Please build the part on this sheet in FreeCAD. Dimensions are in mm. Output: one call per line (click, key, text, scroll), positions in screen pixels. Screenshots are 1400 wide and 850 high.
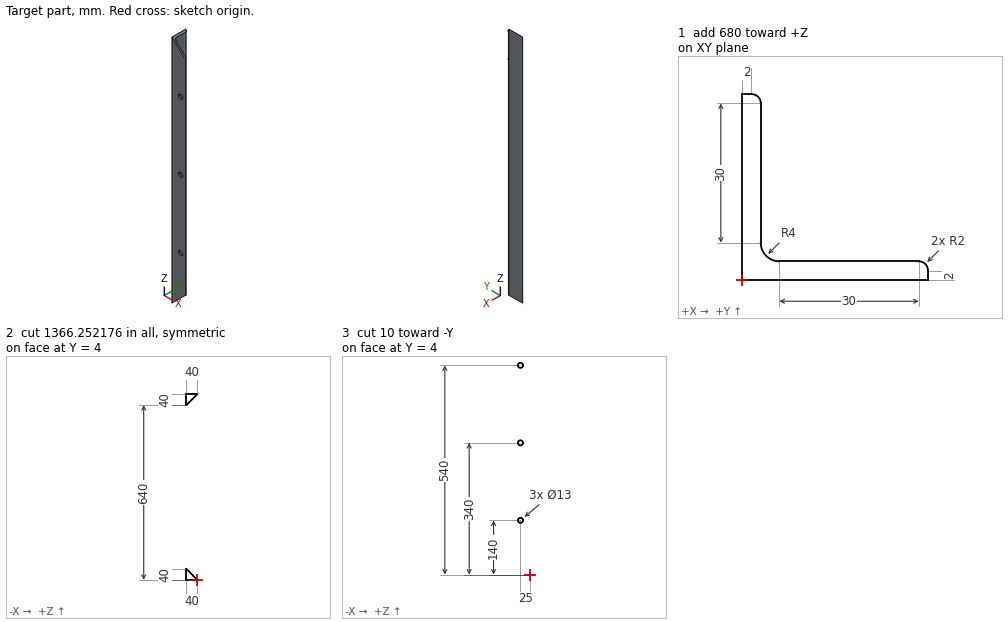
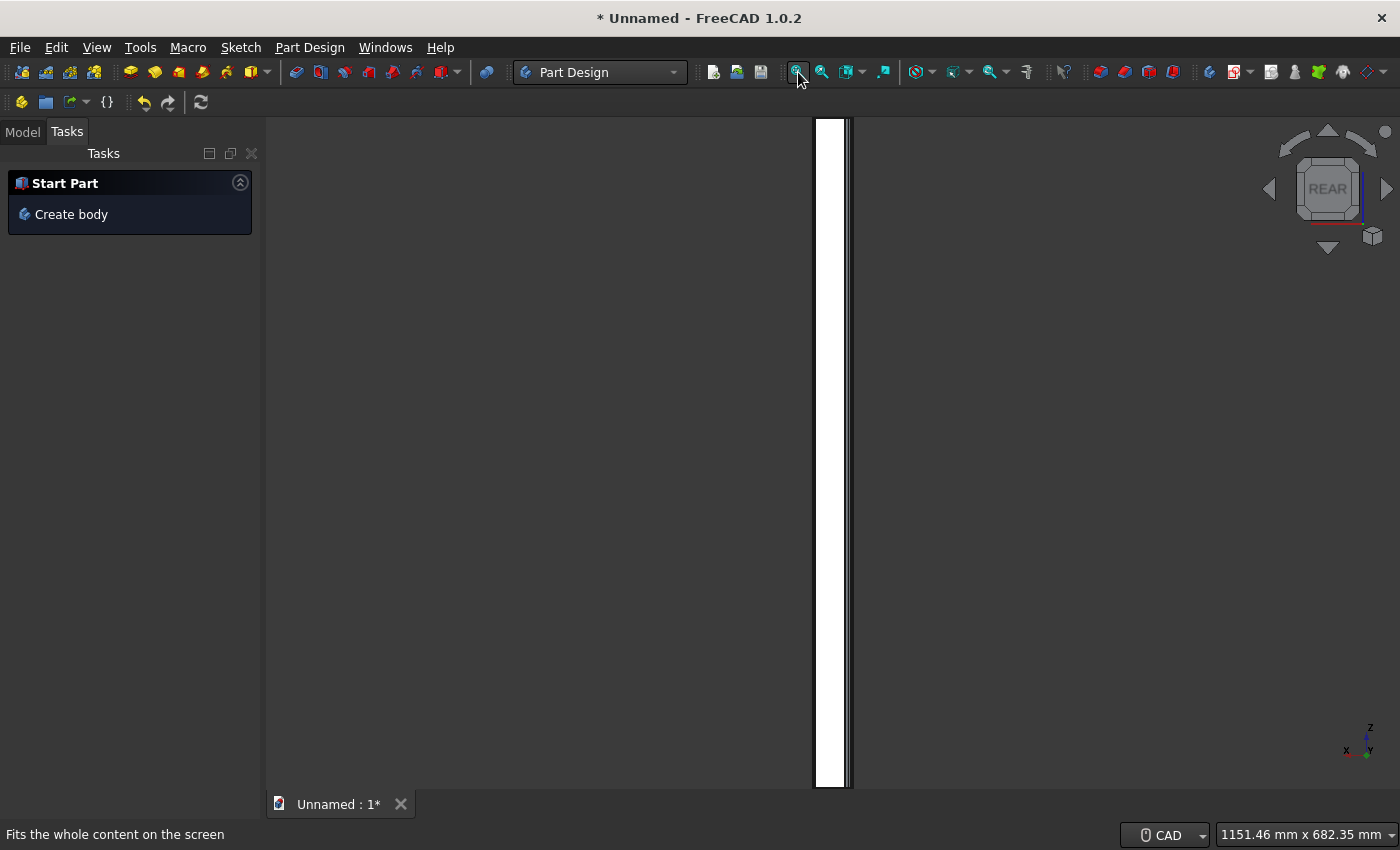
click(830, 165)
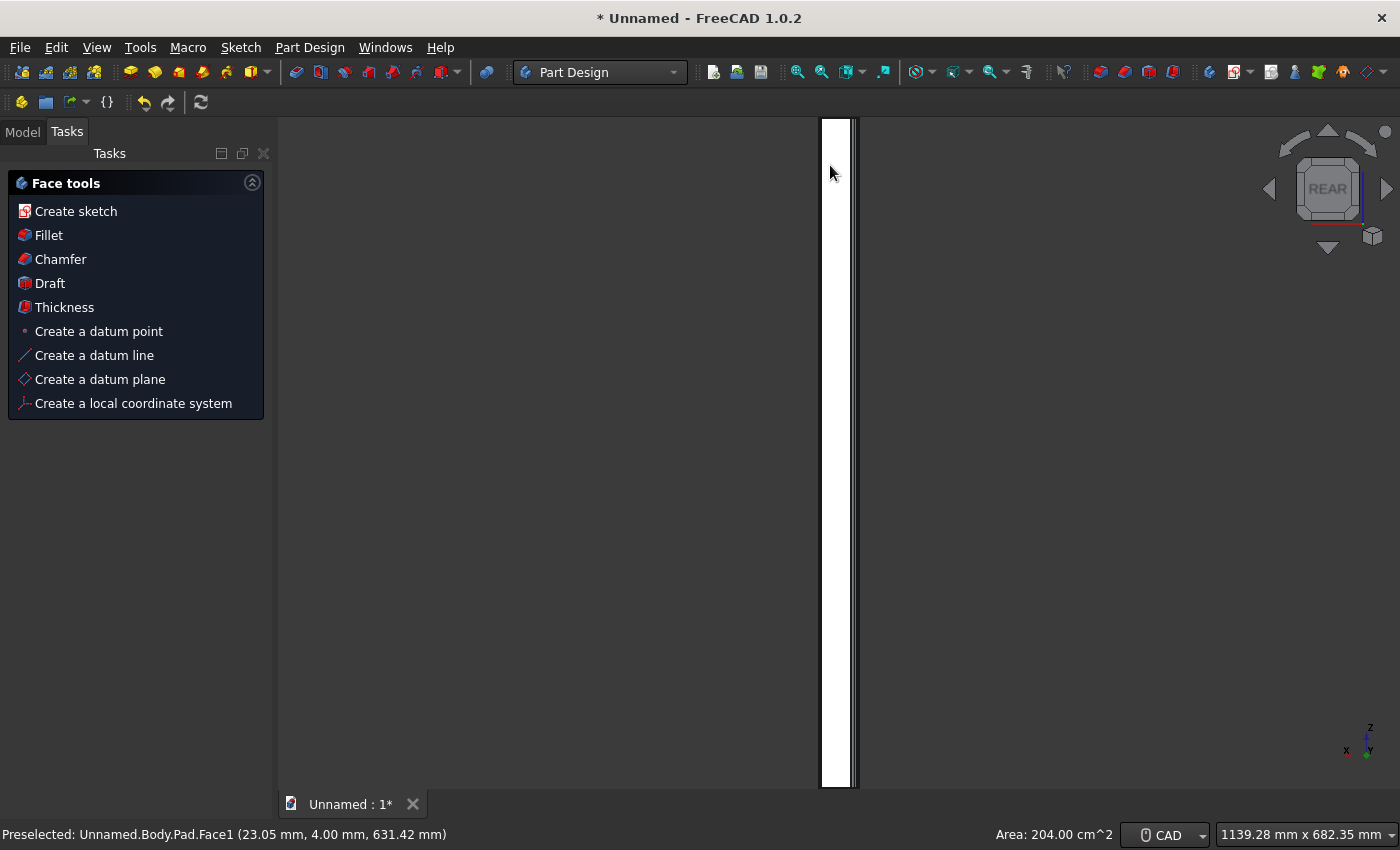
click(1234, 72)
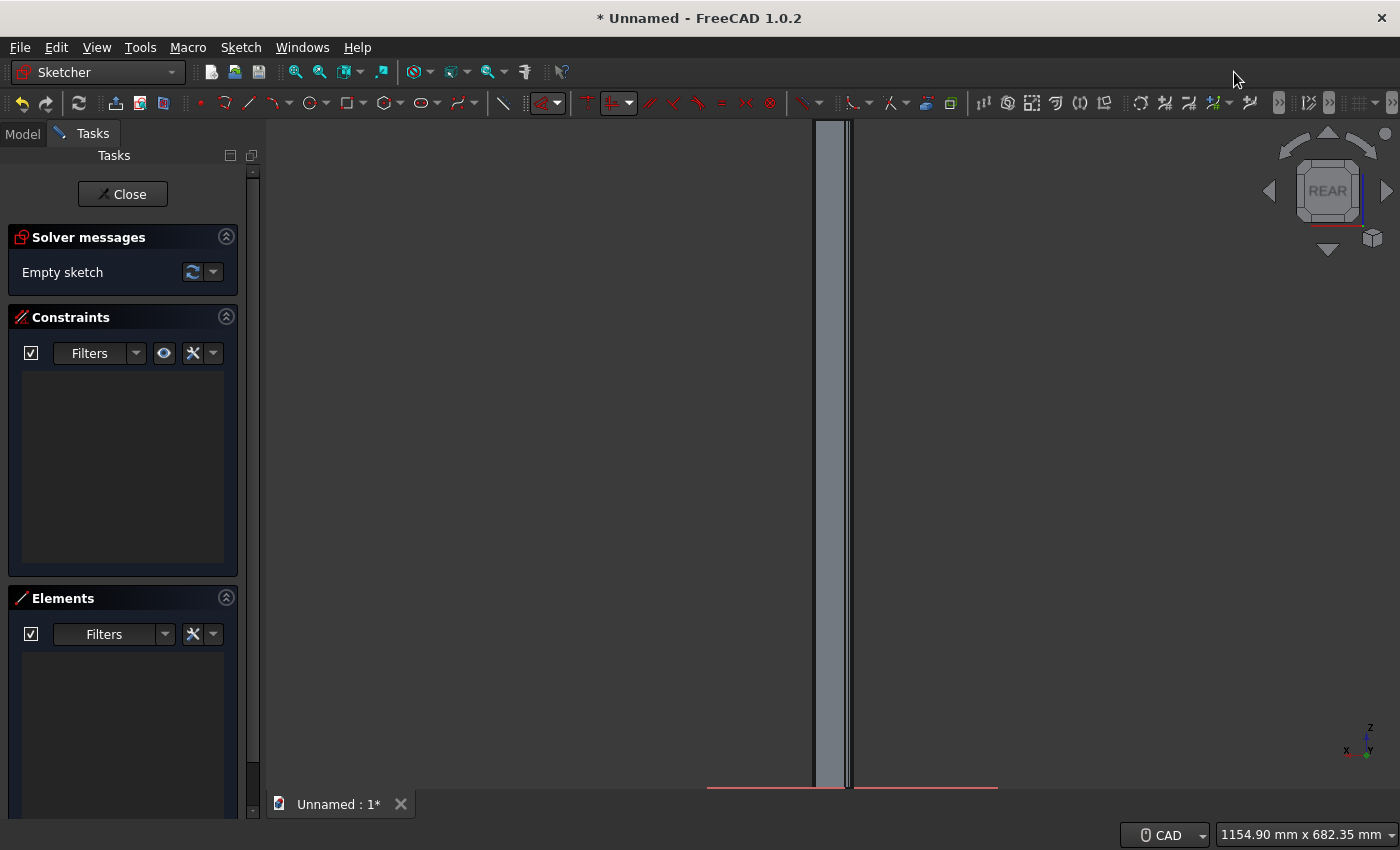
click(164, 104)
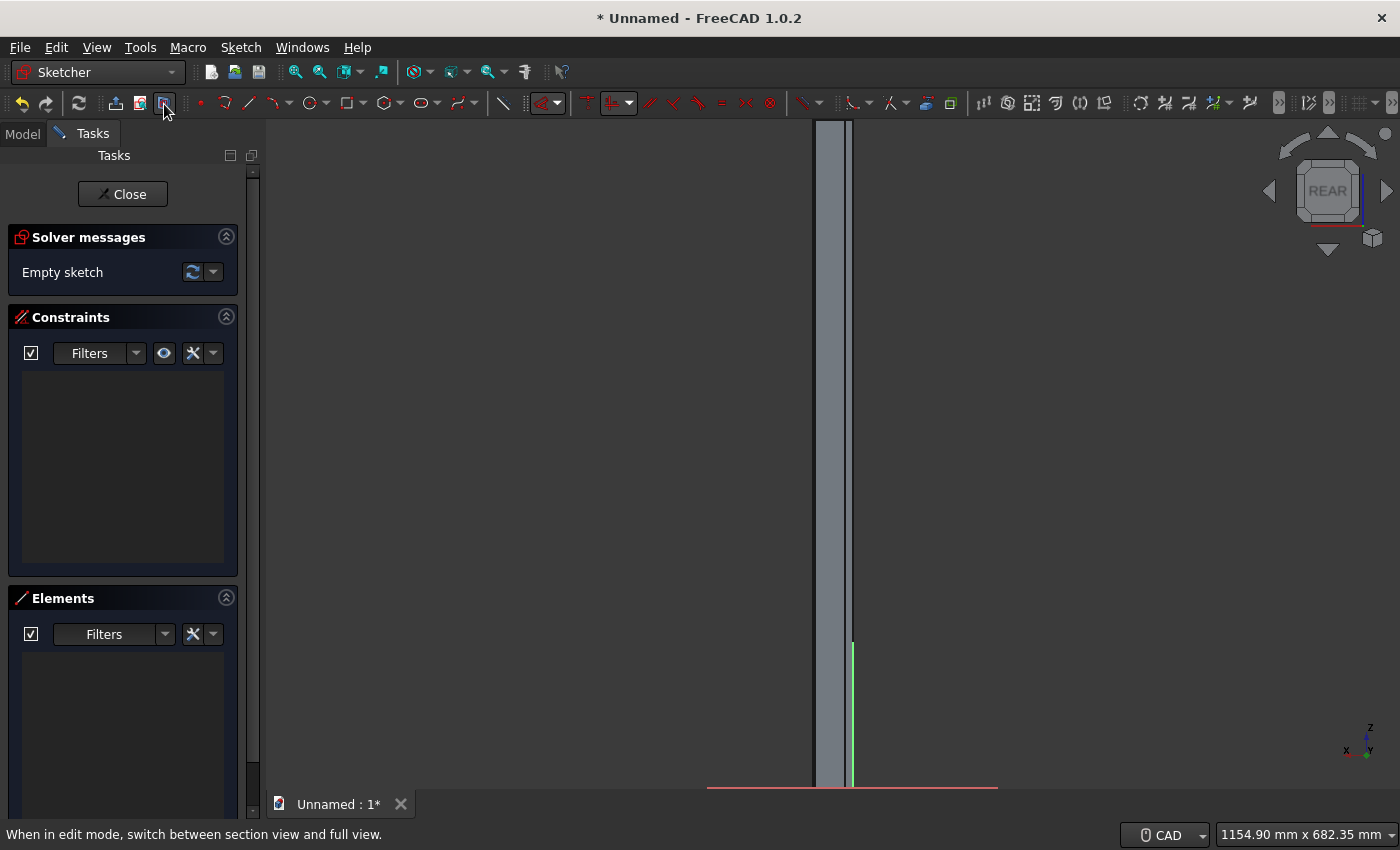
scroll(625, 454, down, 2)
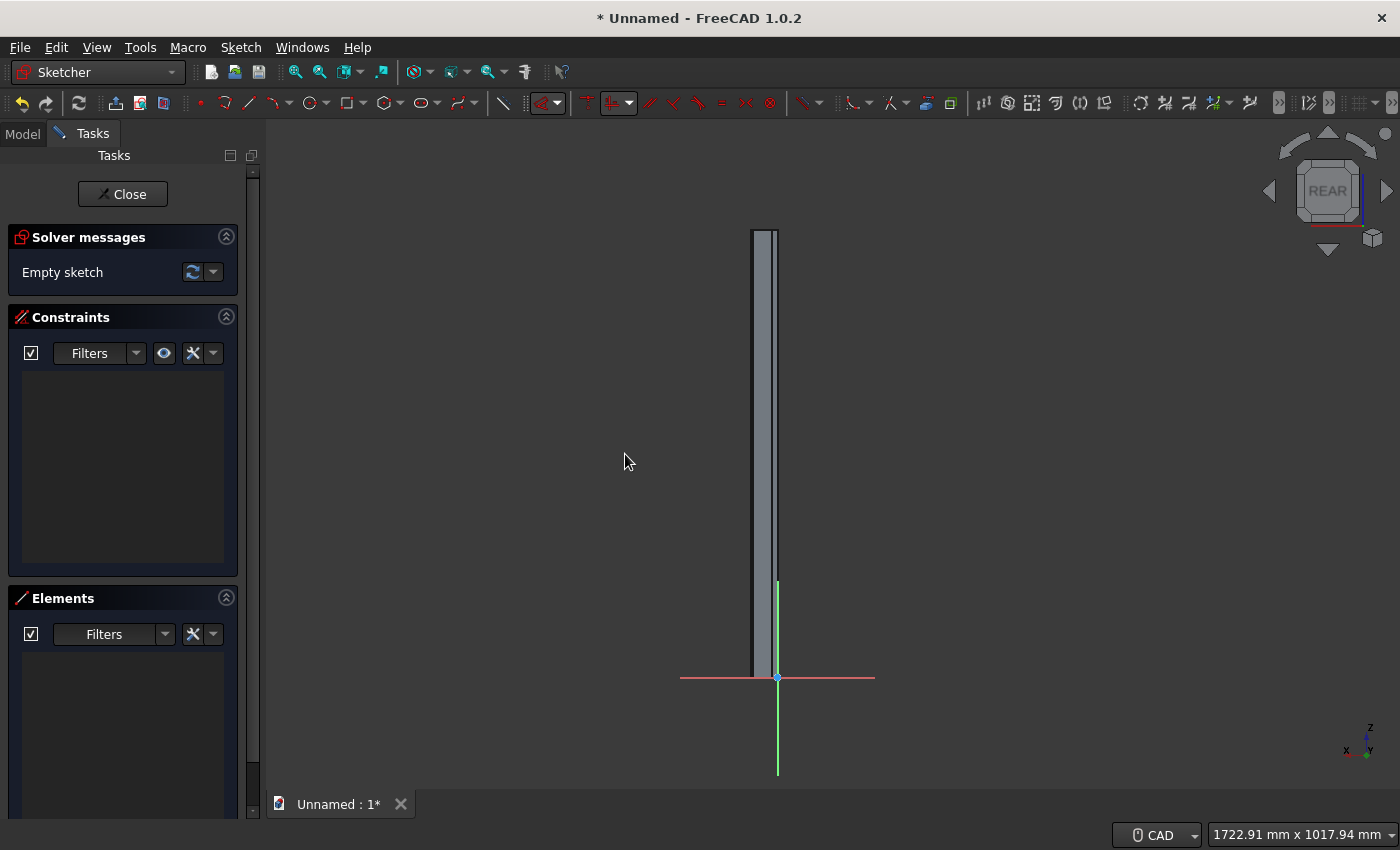
click(226, 104)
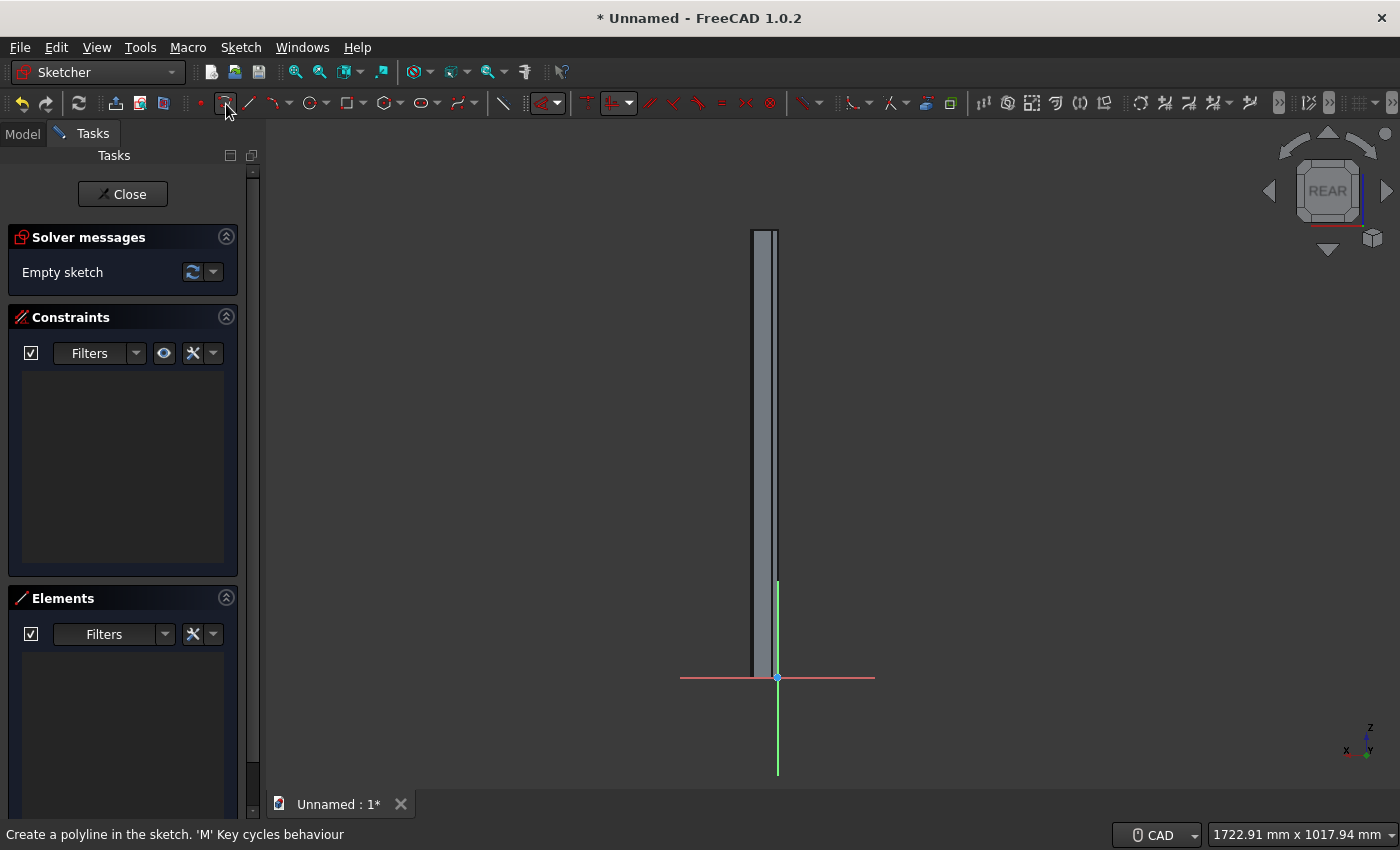
click(778, 678)
click(751, 652)
click(751, 669)
click(778, 678)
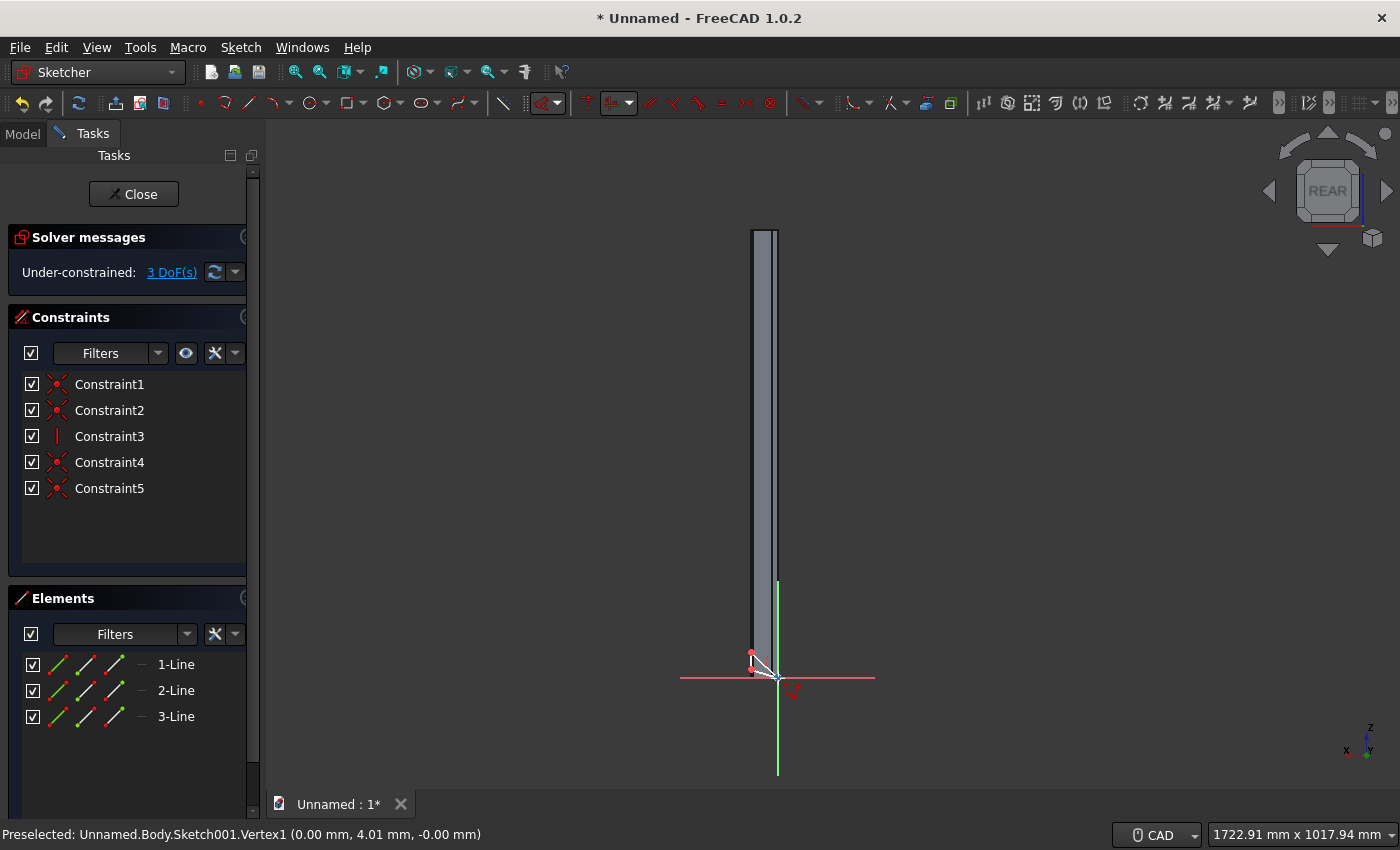
click(751, 257)
click(778, 230)
click(751, 230)
click(751, 258)
key(Escape)
key(Escape)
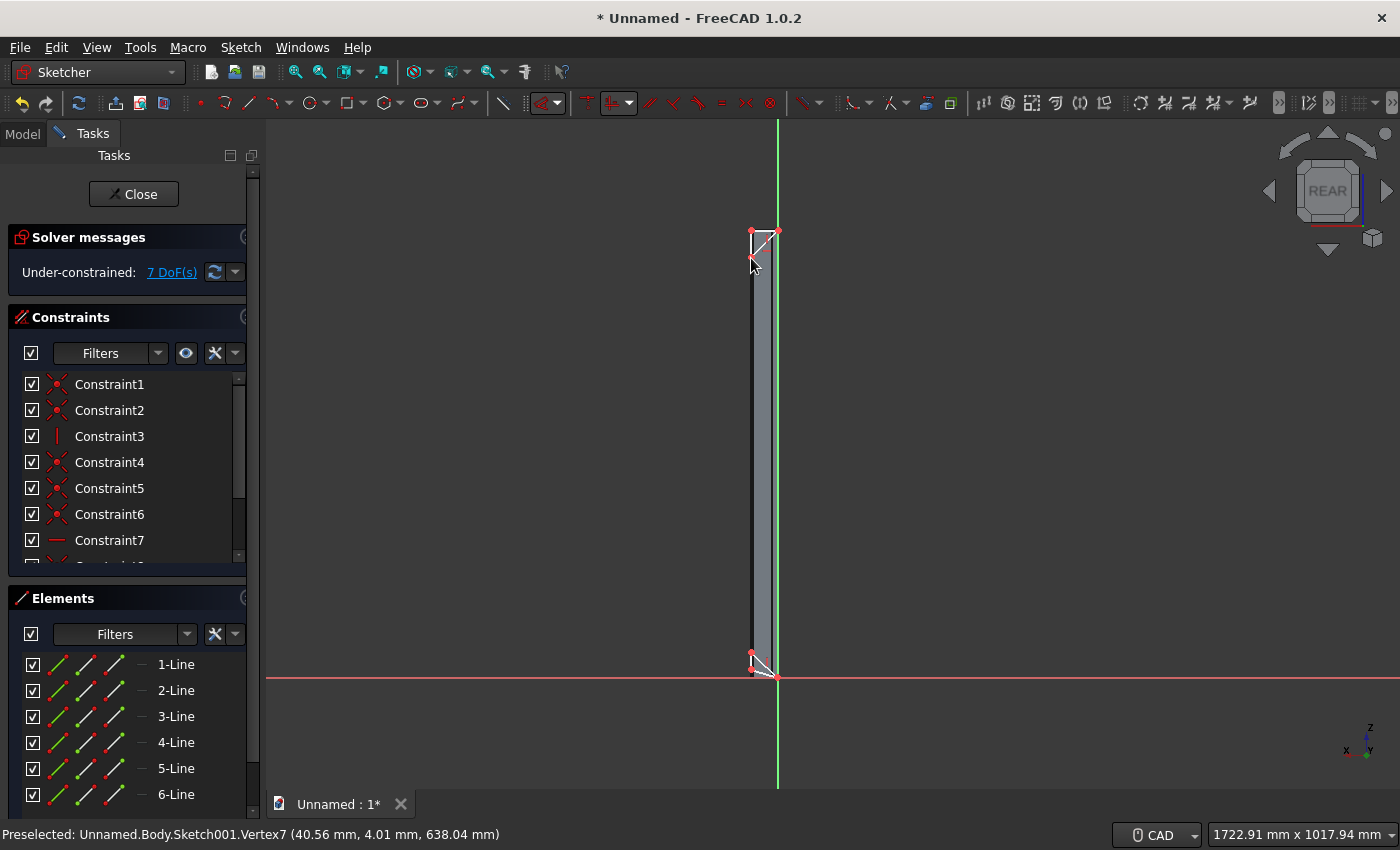
scroll(764, 674, up, 4)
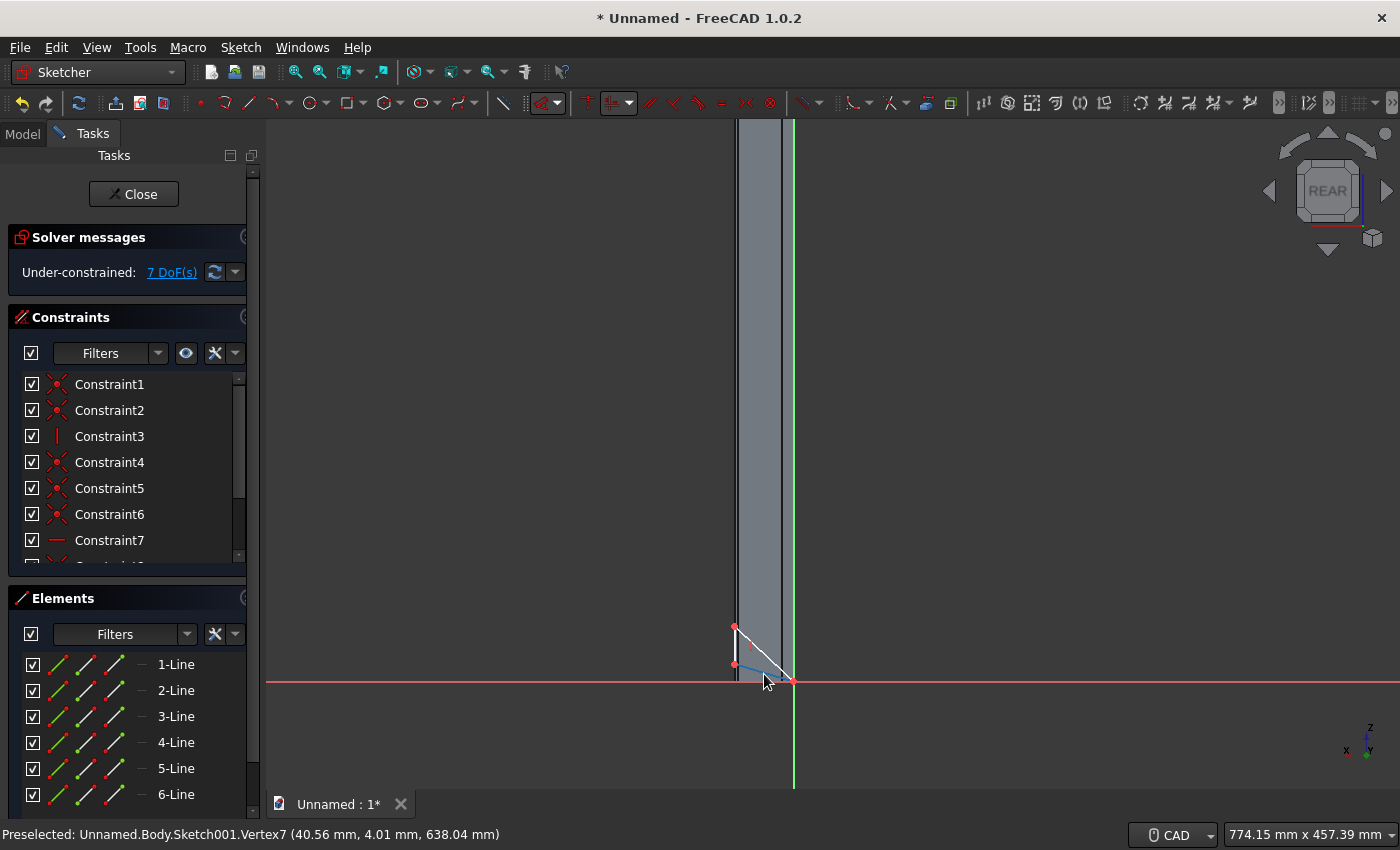
click(764, 673)